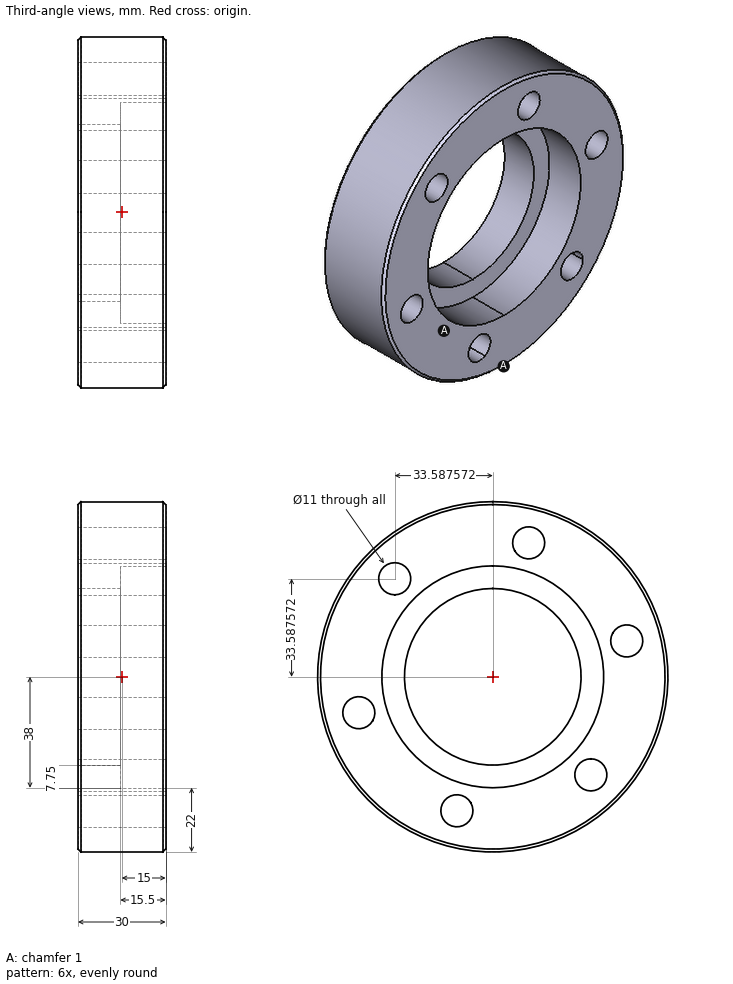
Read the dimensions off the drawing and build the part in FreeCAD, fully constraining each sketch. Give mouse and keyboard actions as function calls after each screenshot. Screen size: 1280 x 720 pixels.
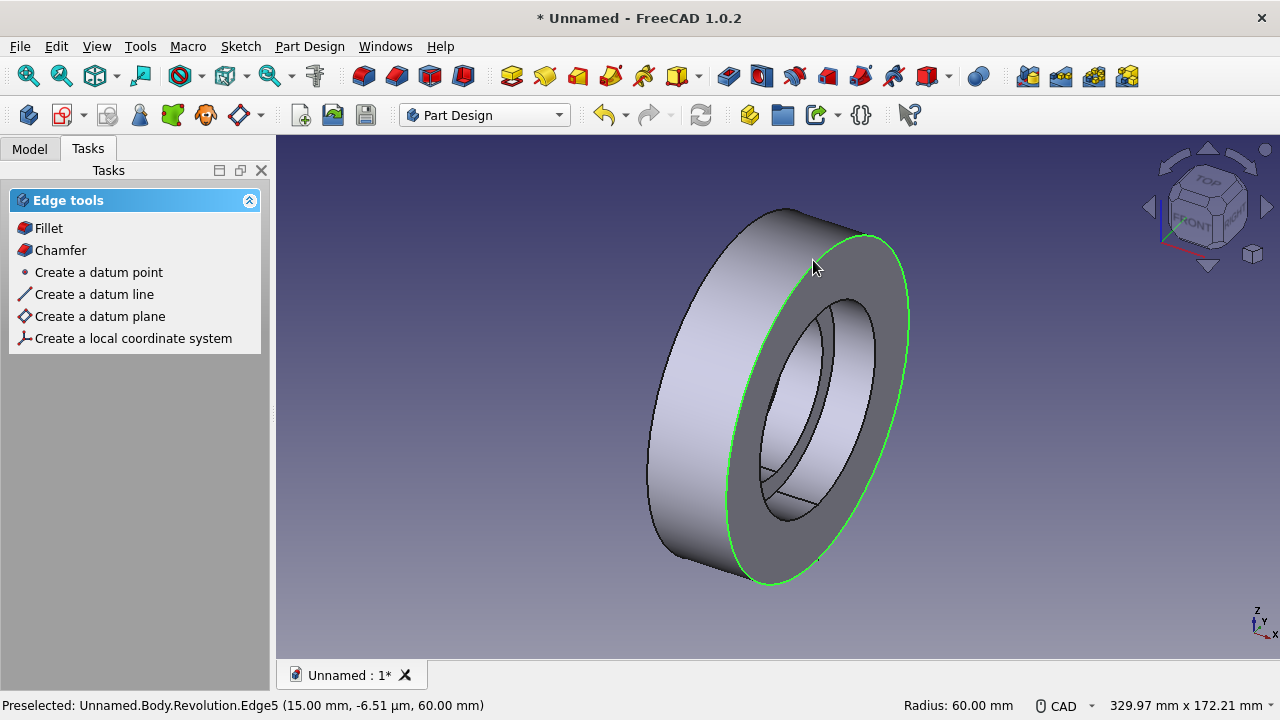
key(0)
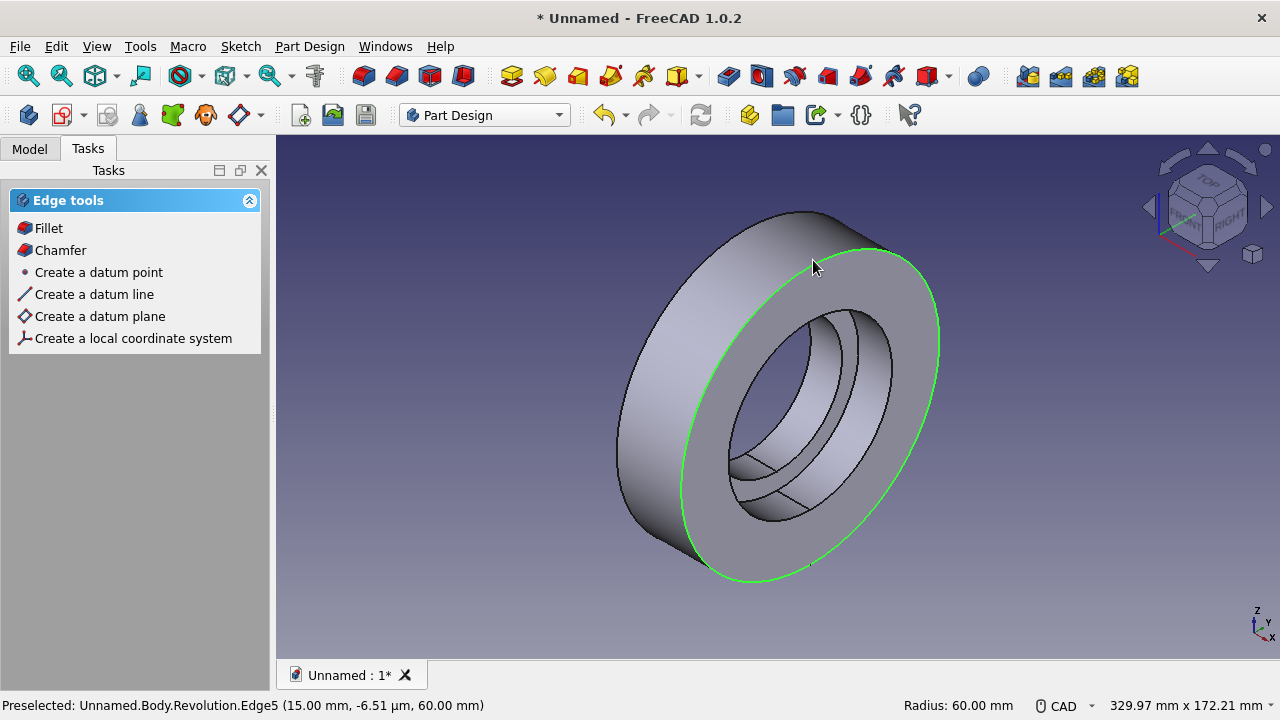
key(2)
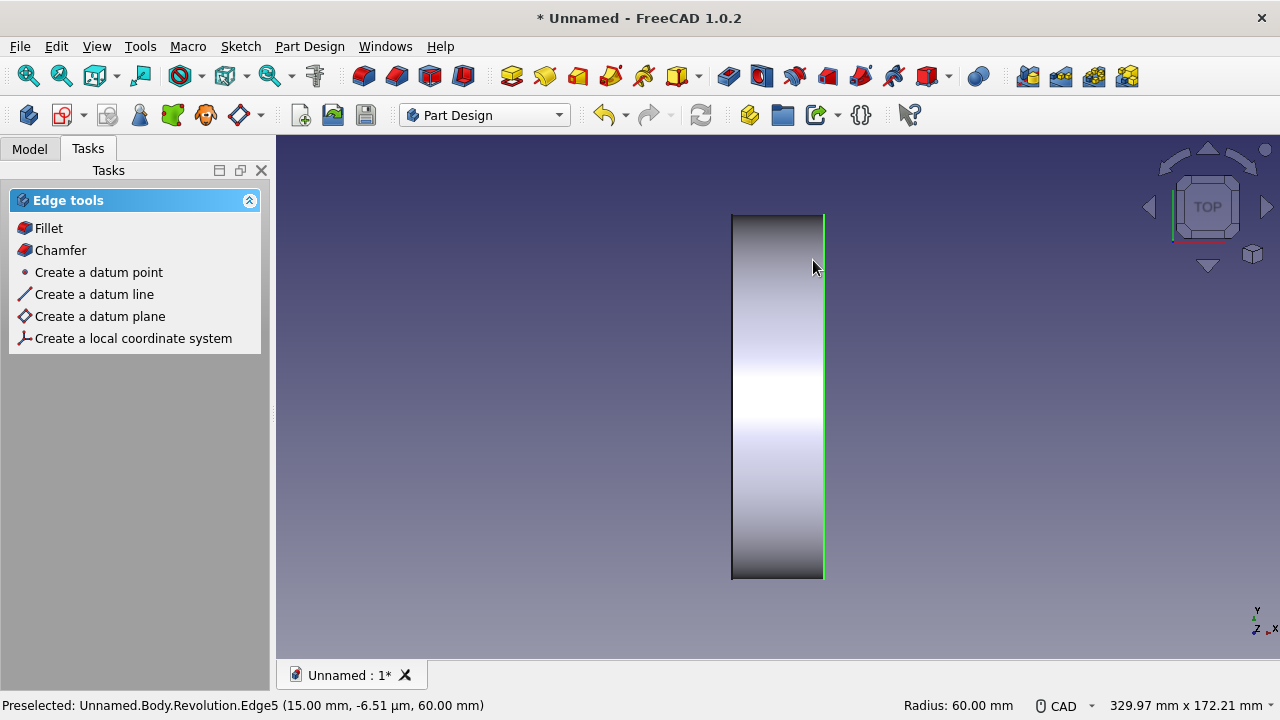
click(732, 396, ctrl)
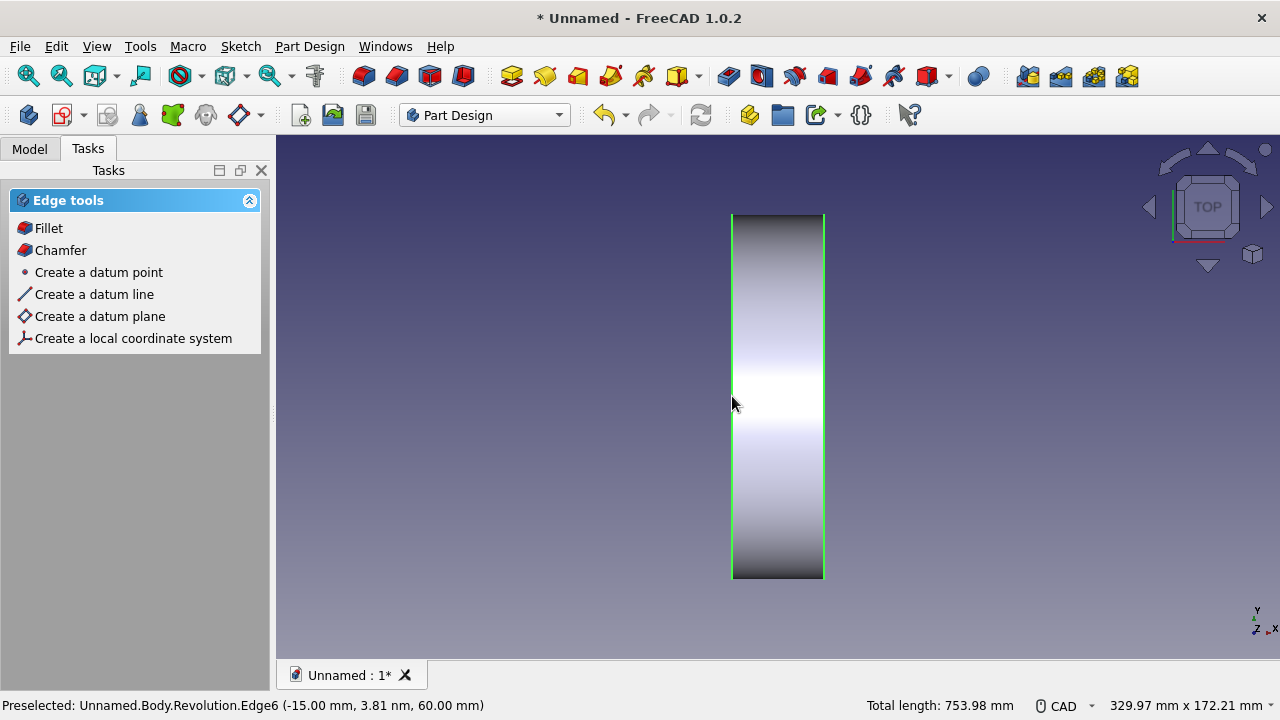
click(397, 76)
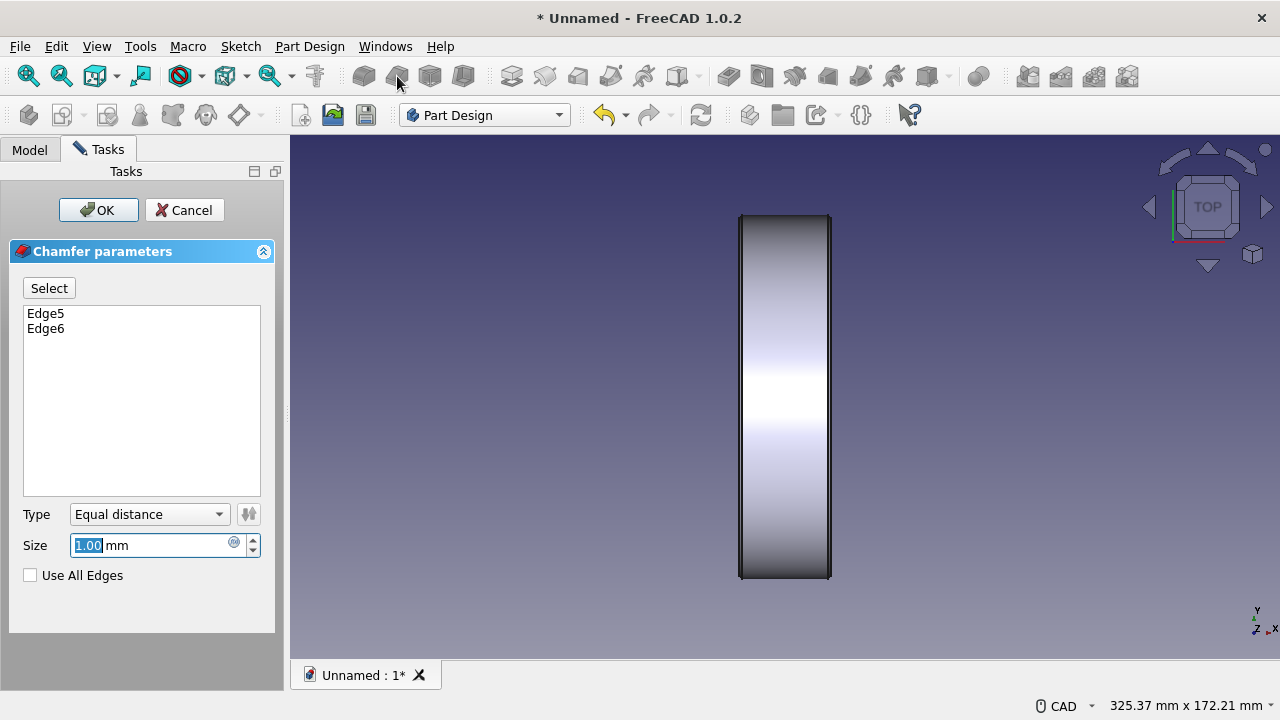
text(1)
key(Tab)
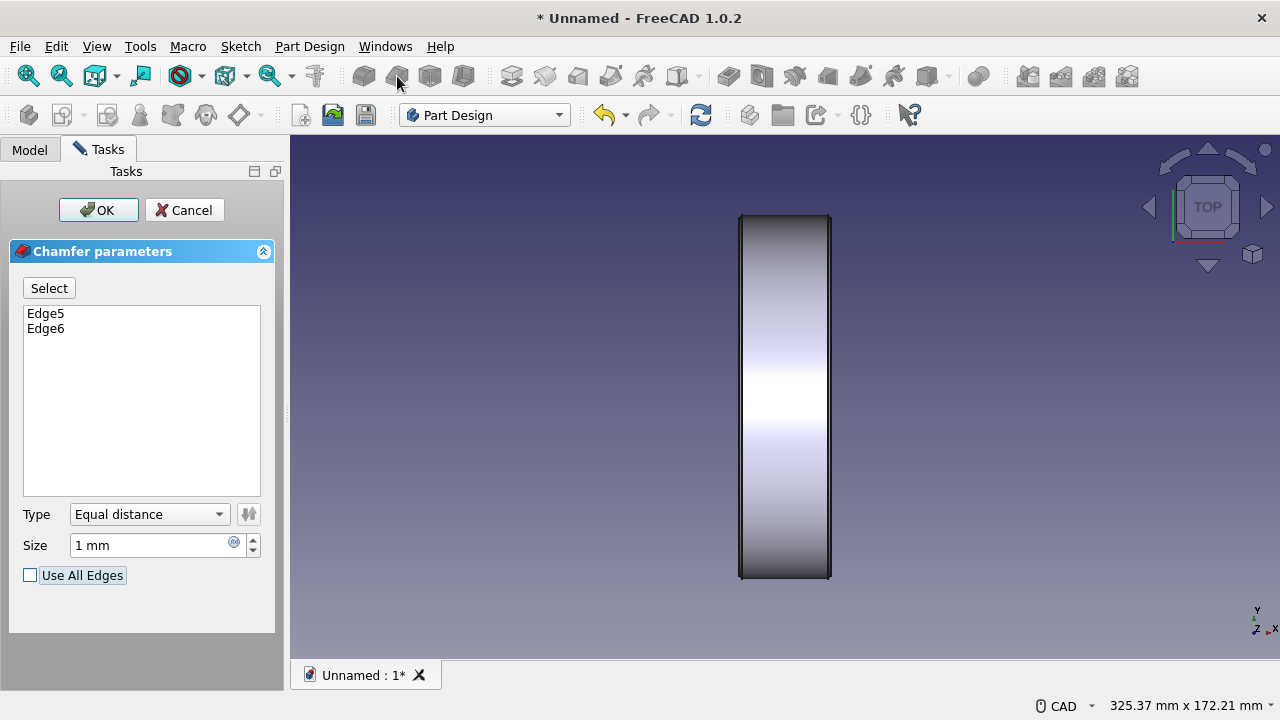
click(99, 210)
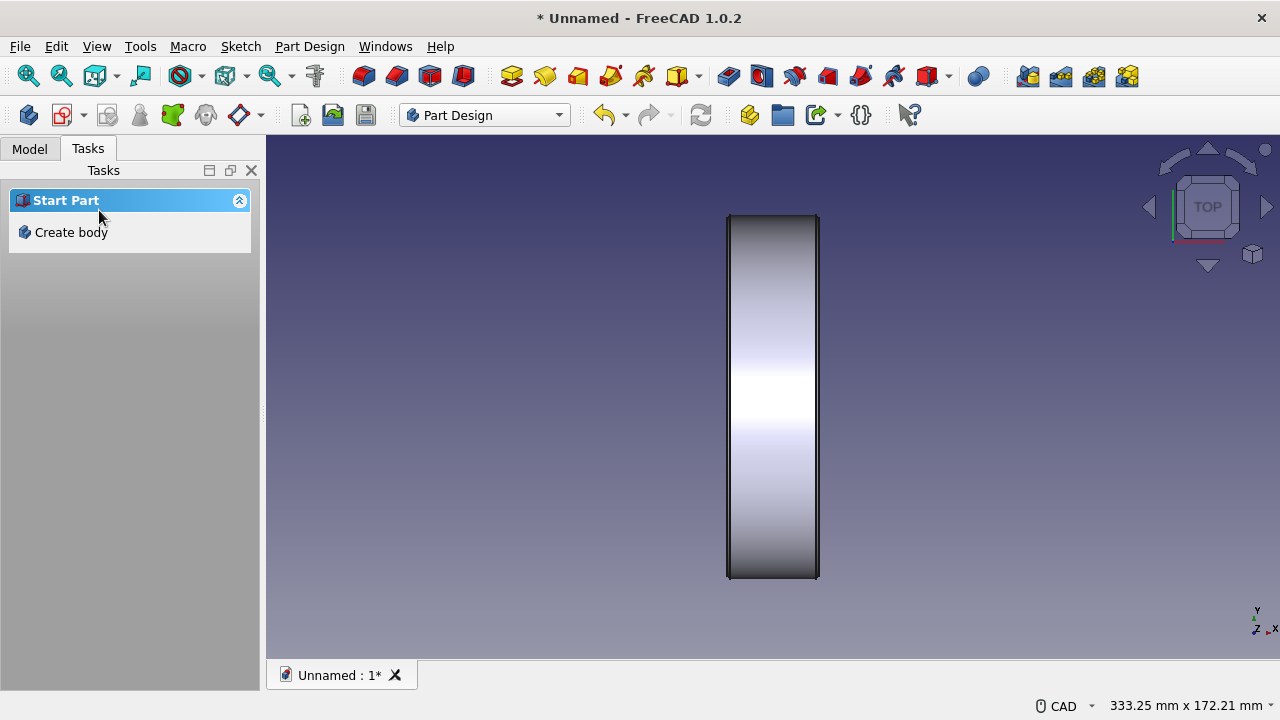
key(6)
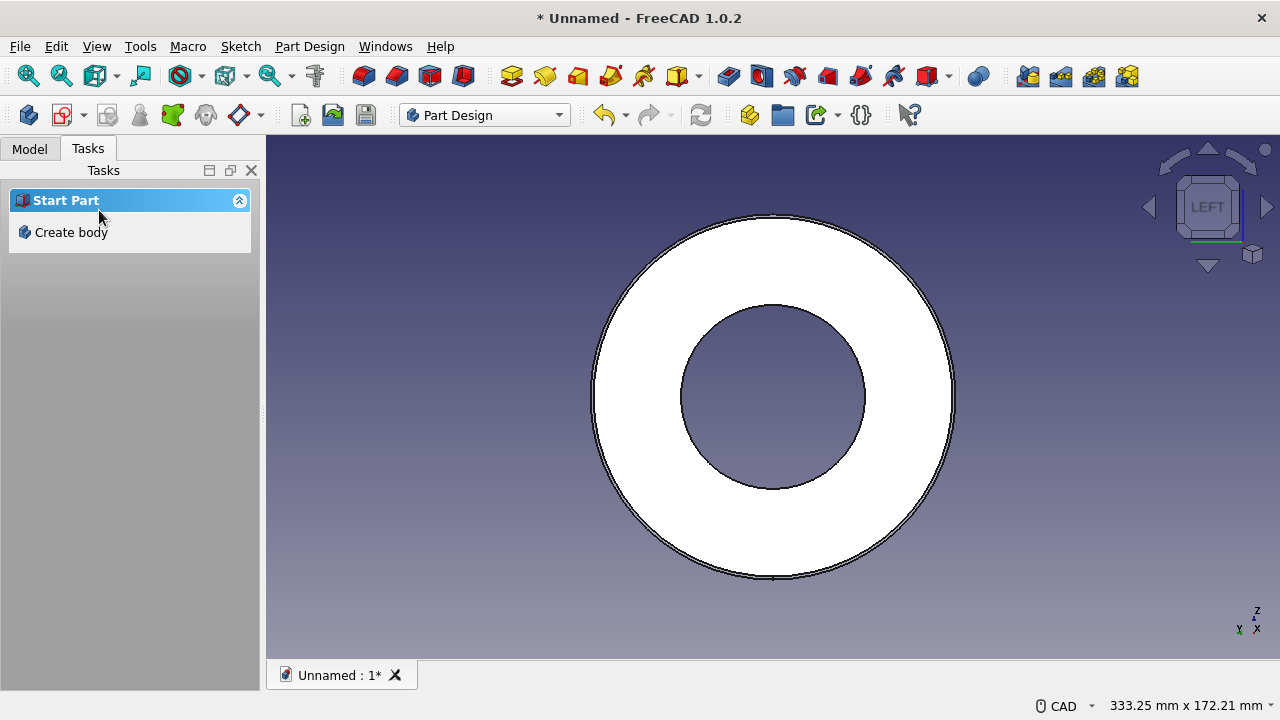
click(670, 499)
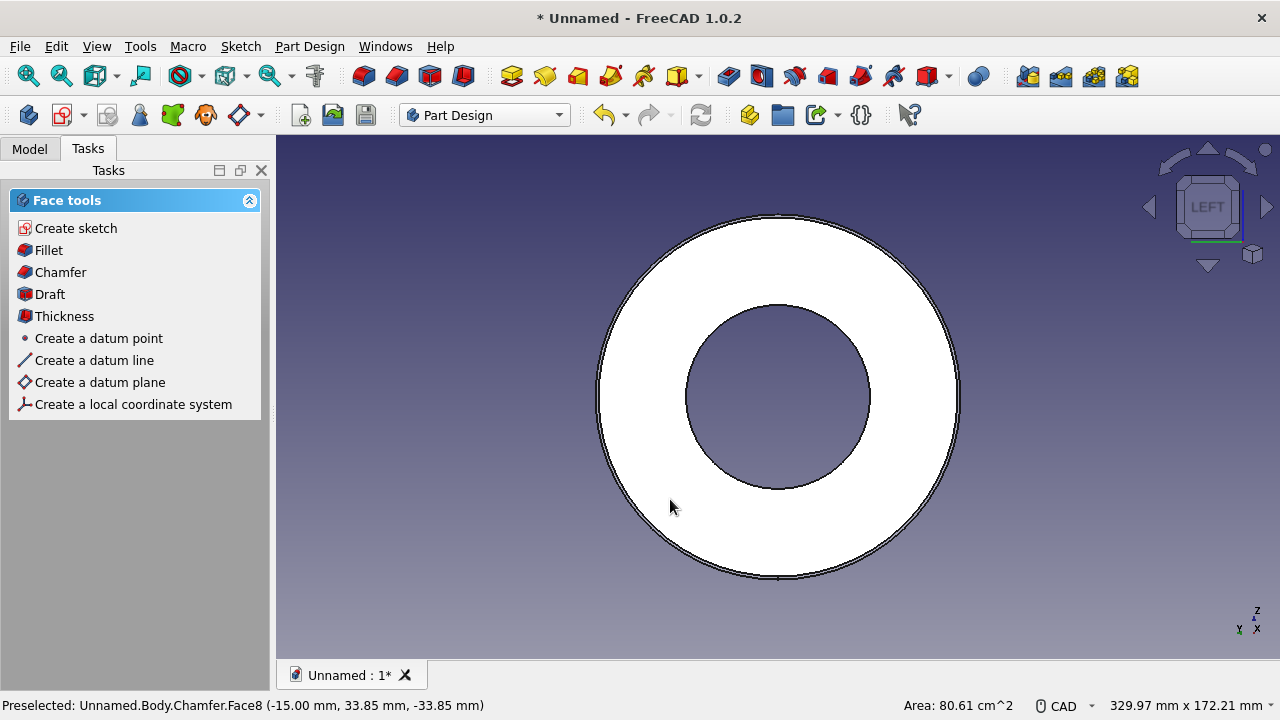
click(62, 116)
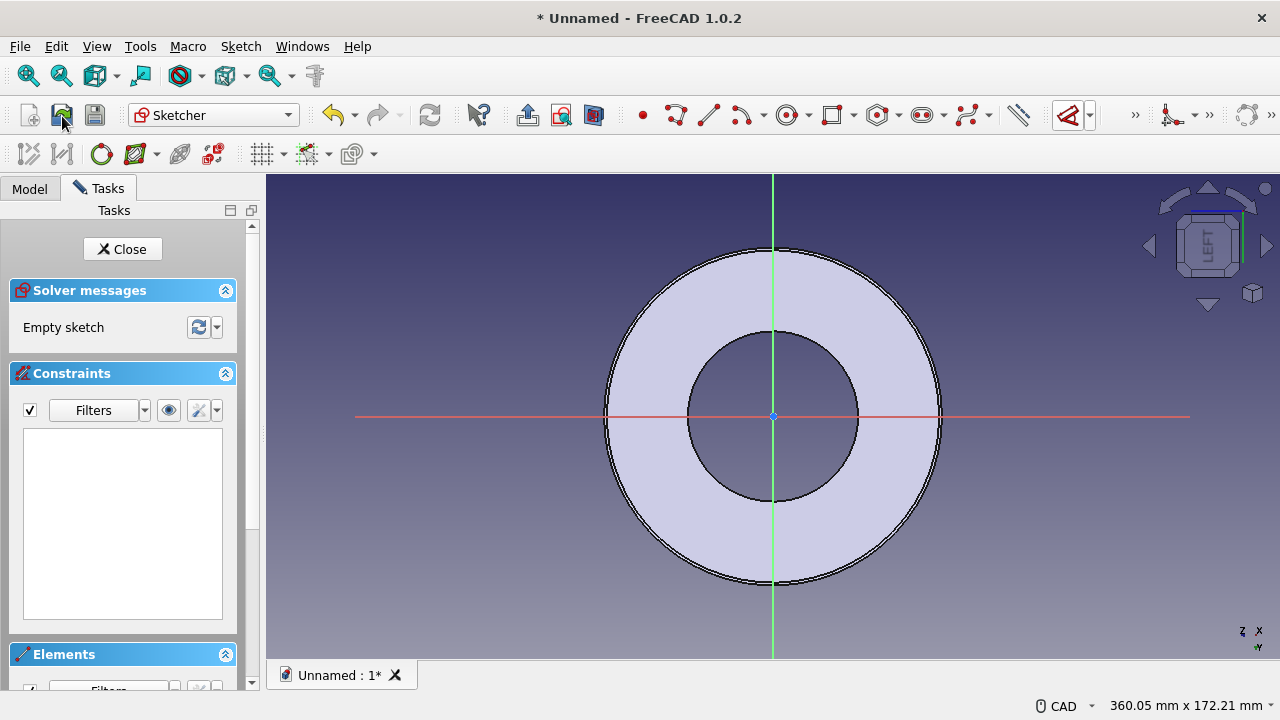
scroll(675, 310, up, 11)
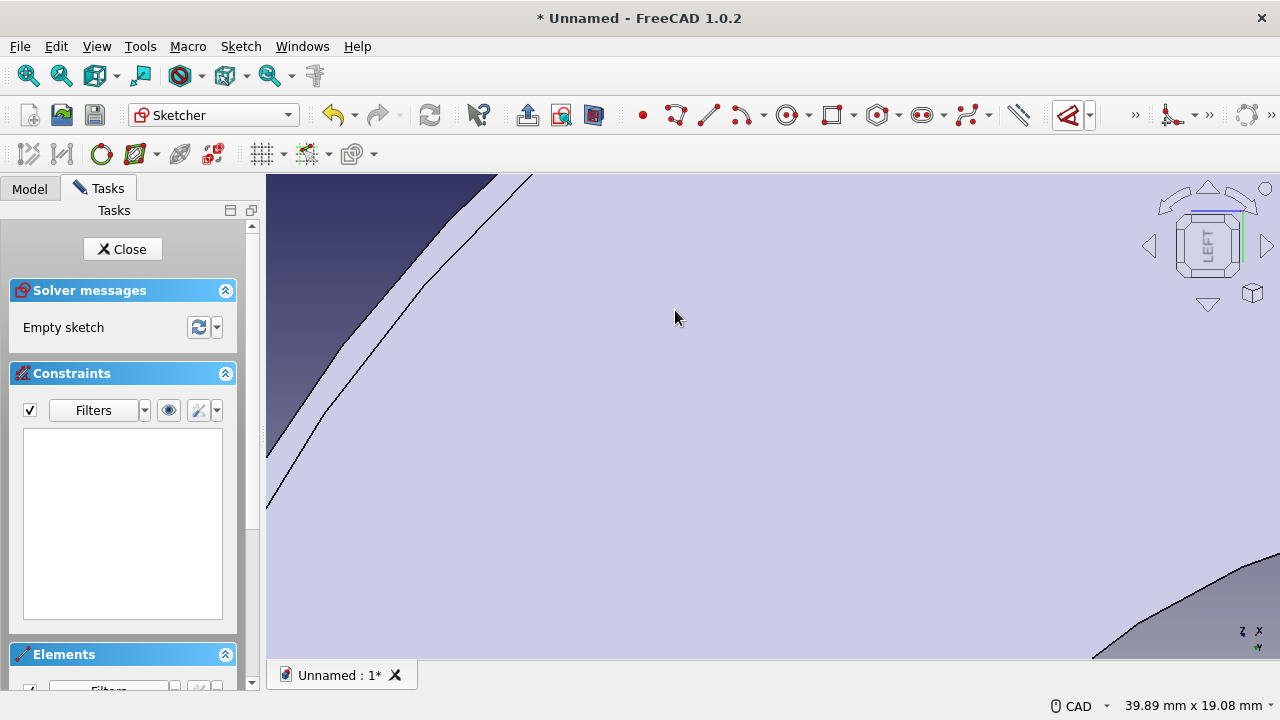
key(g)
key(c)